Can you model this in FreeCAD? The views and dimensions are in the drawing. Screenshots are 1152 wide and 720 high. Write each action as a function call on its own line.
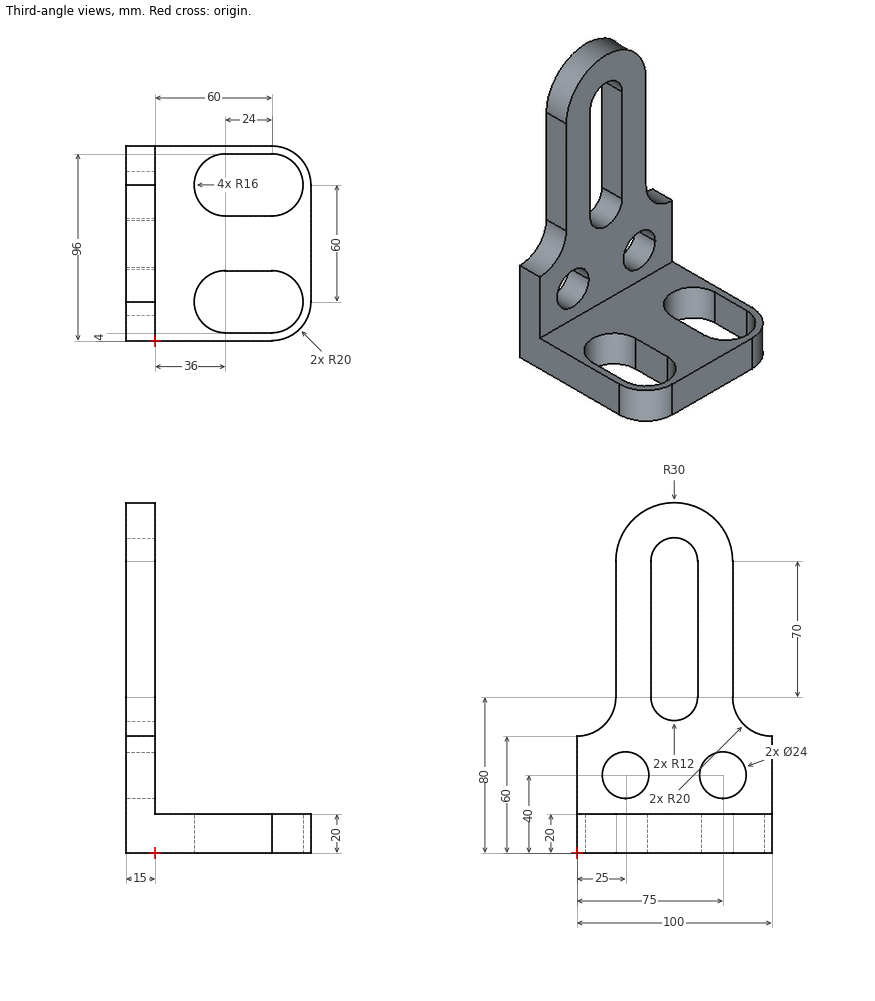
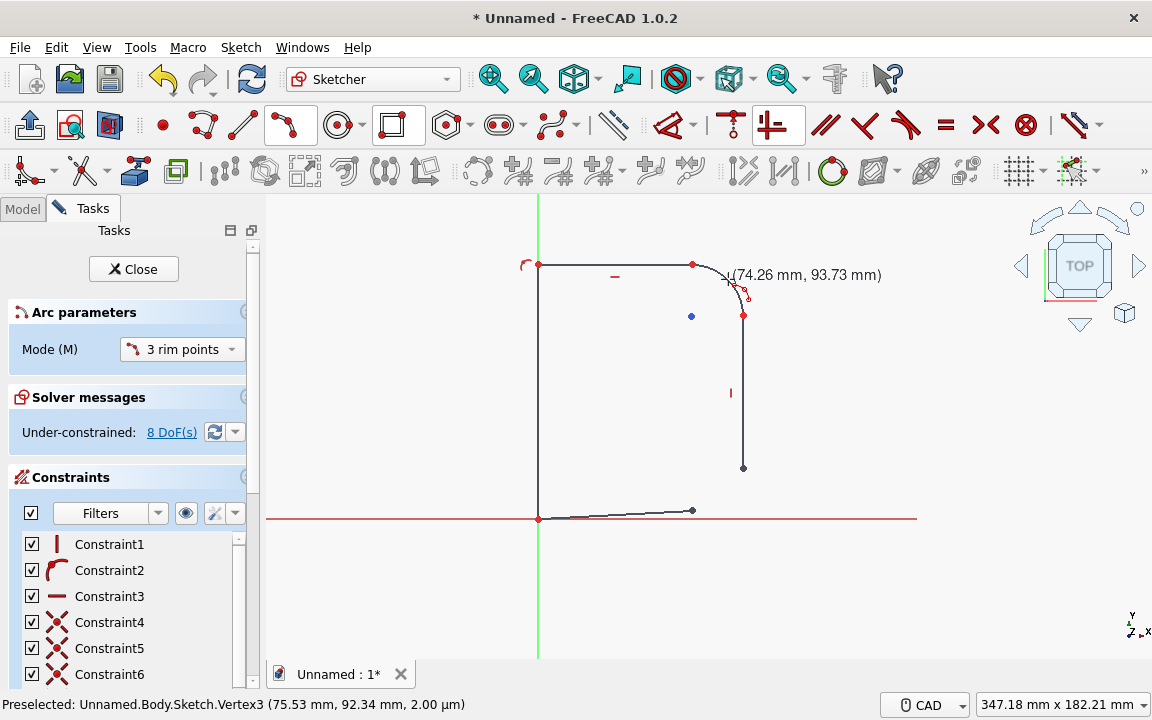
click(692, 511)
click(743, 469)
click(728, 504)
key(Escape)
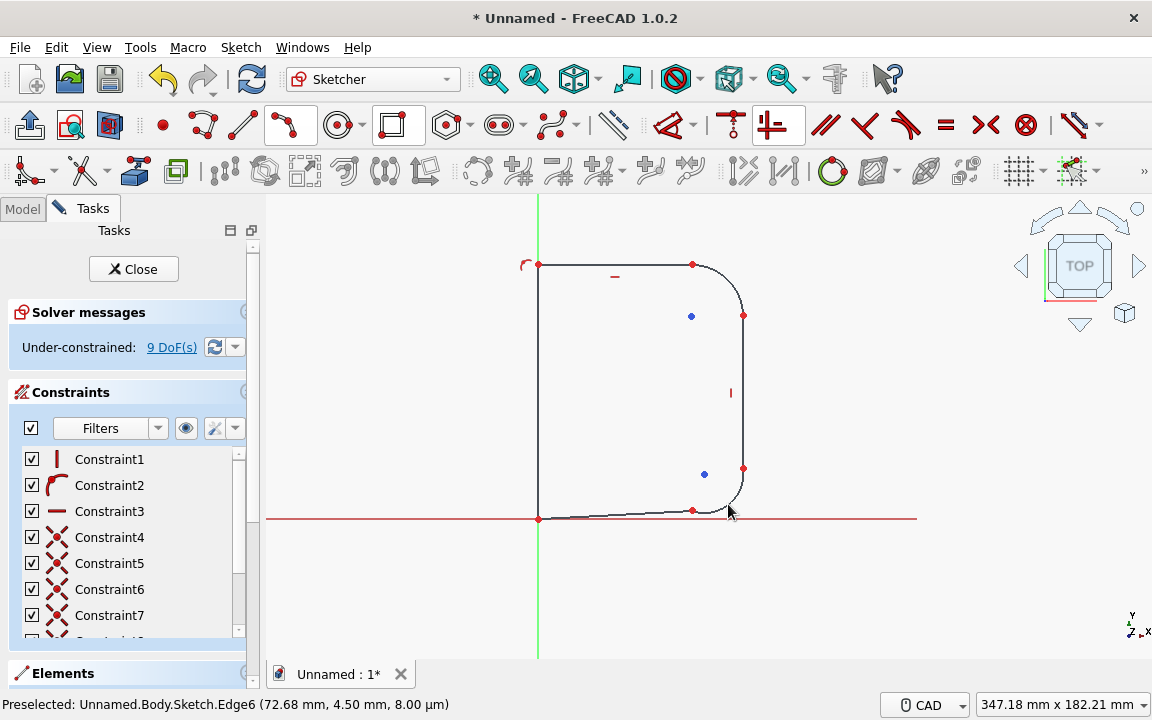
click(743, 423)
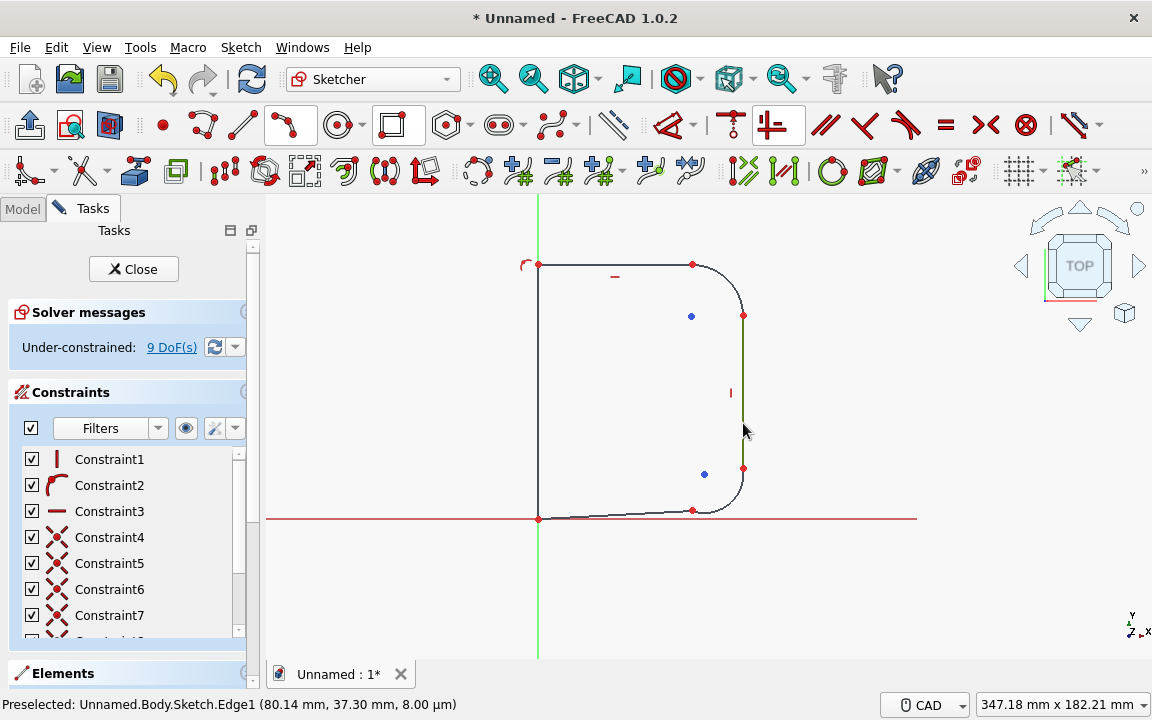
click(737, 293)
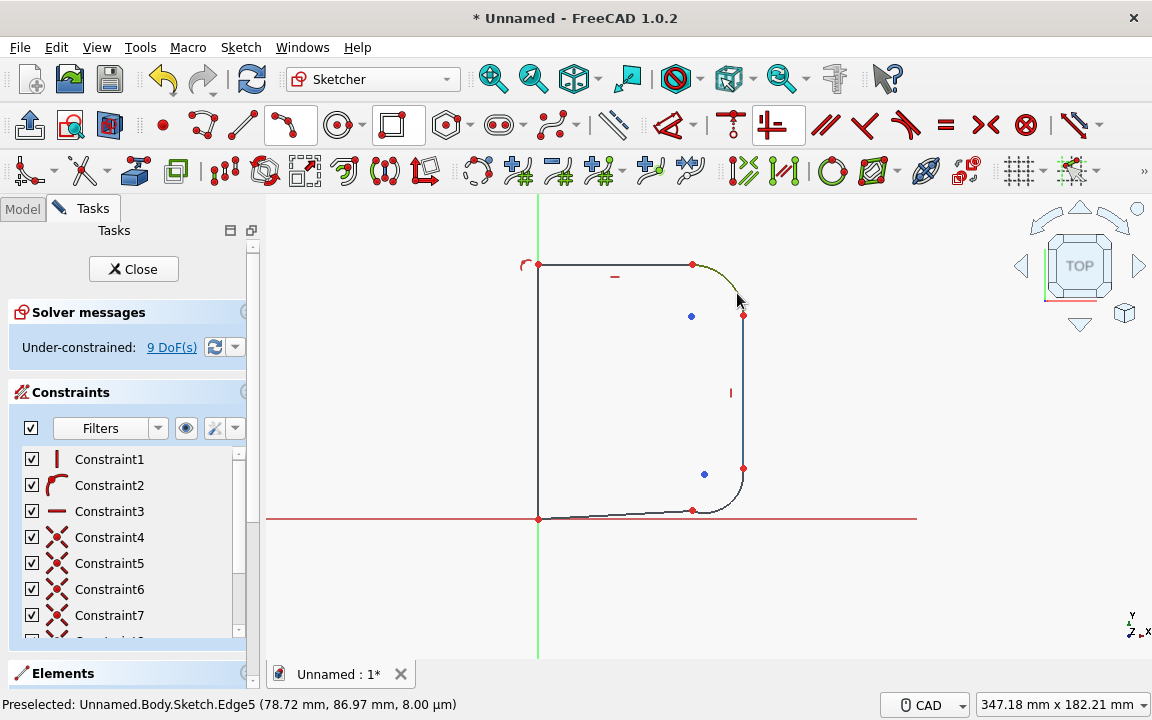
click(906, 126)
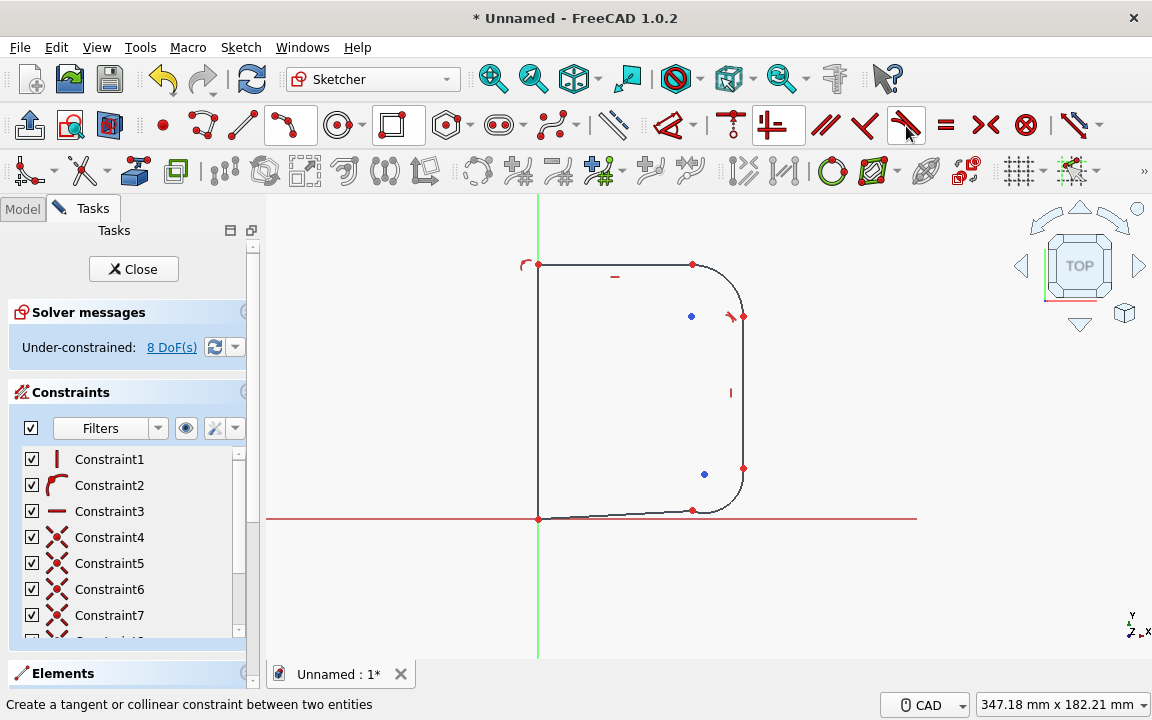
click(743, 423)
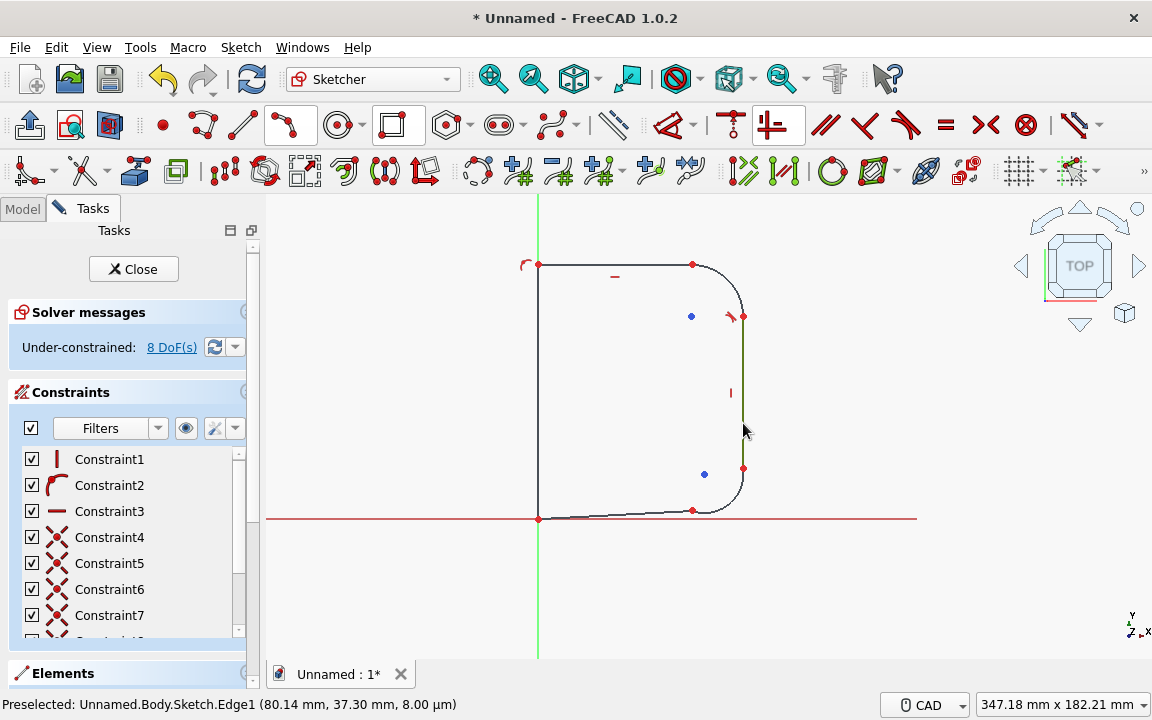
click(739, 492)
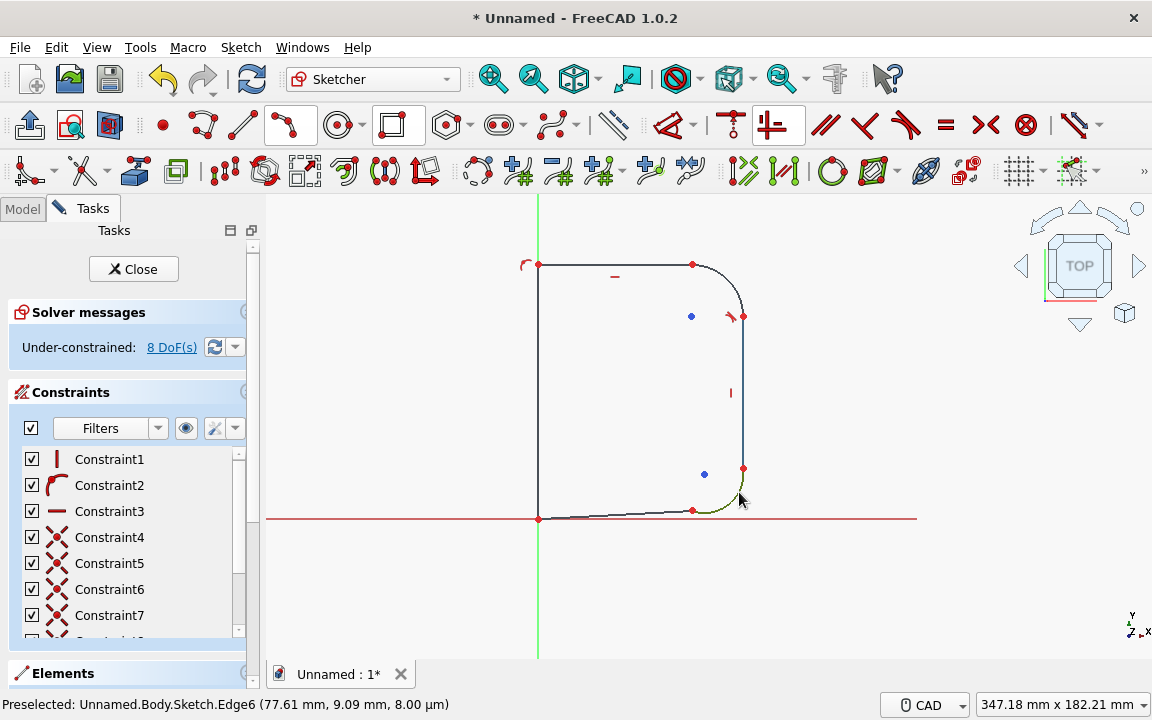
click(906, 126)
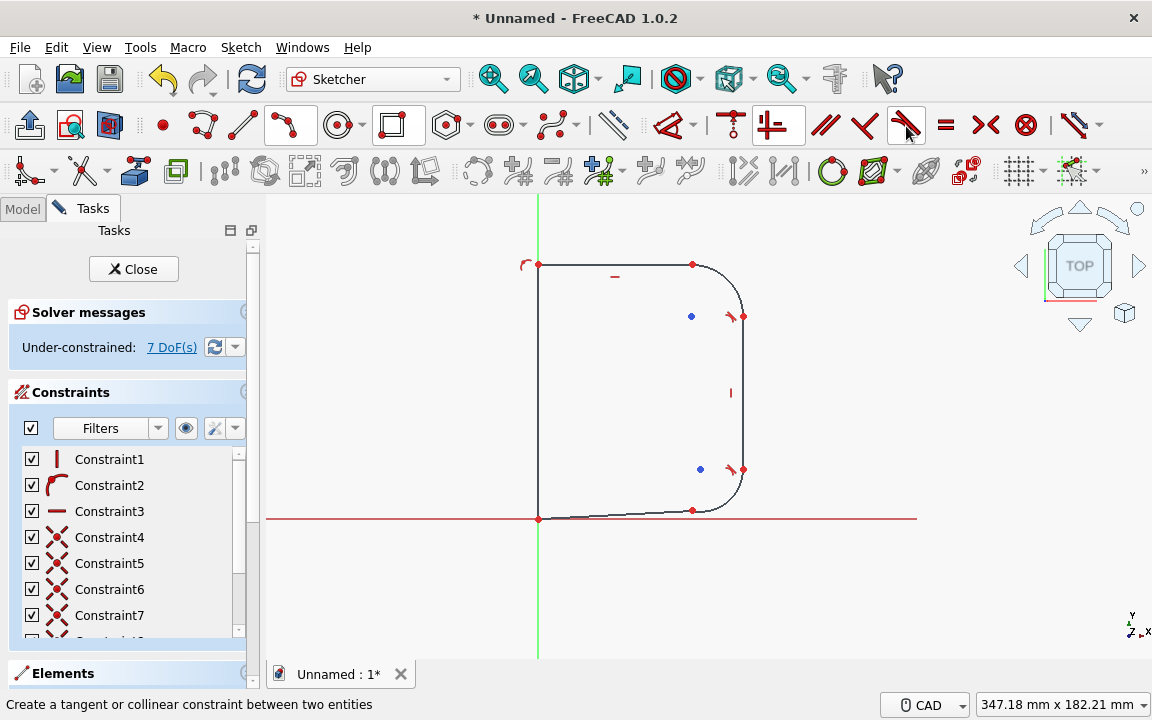
click(646, 265)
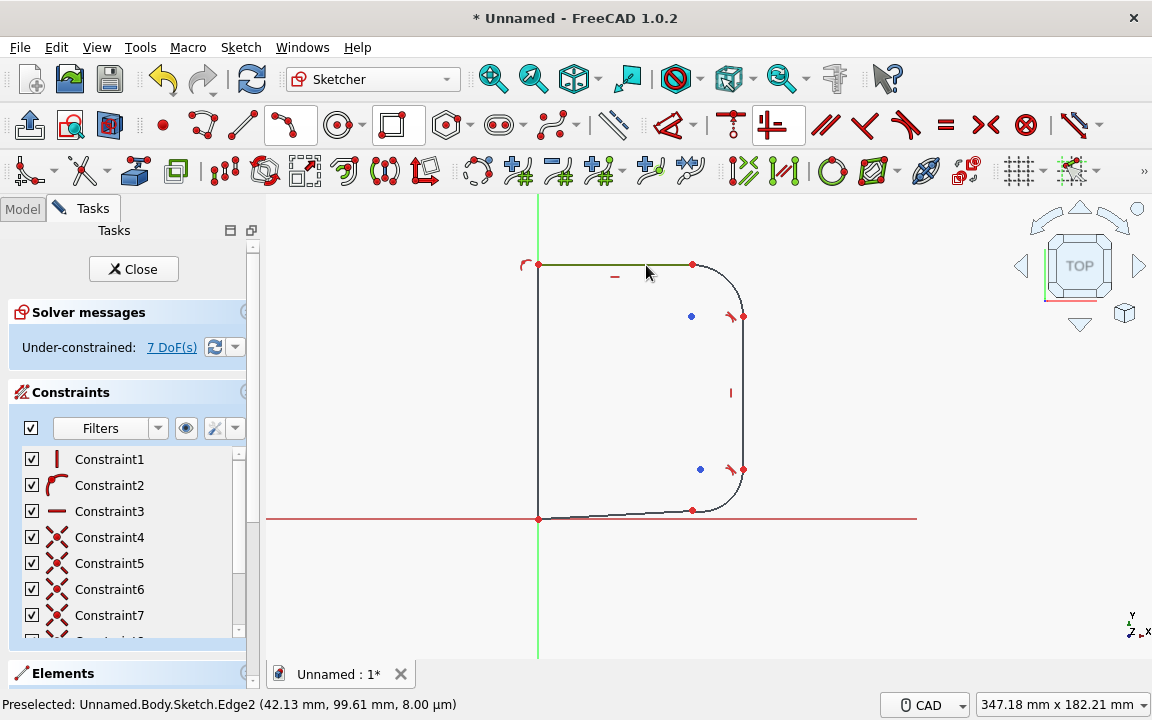
click(737, 293)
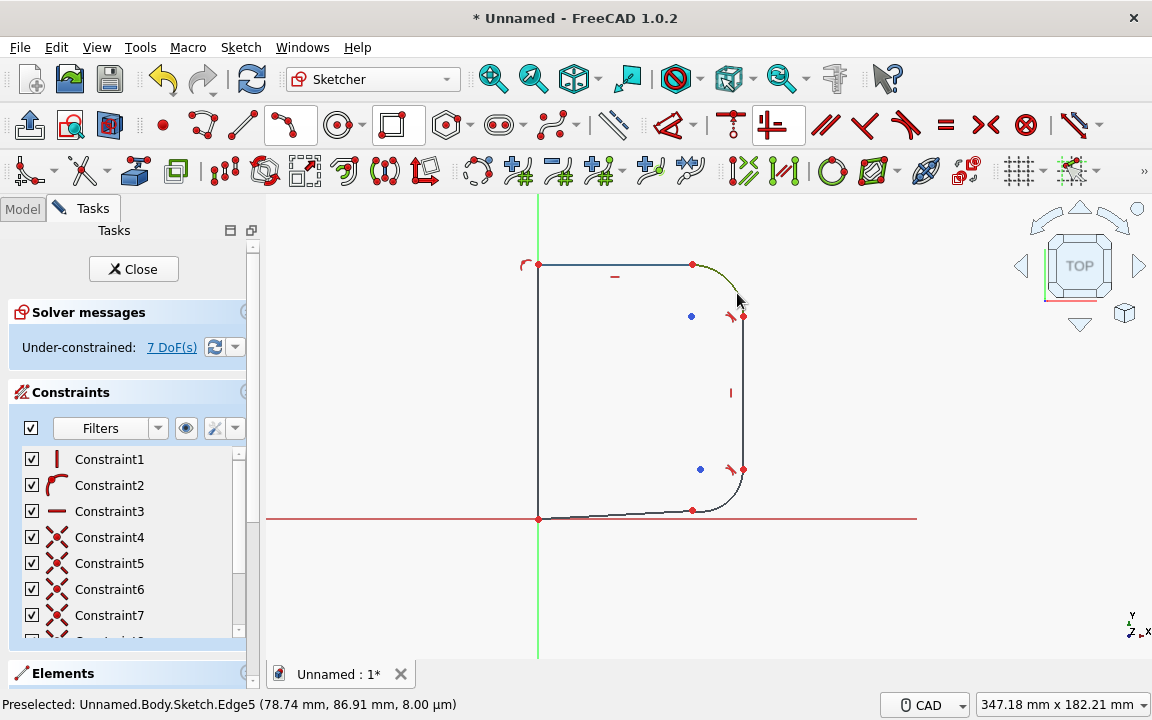
click(906, 126)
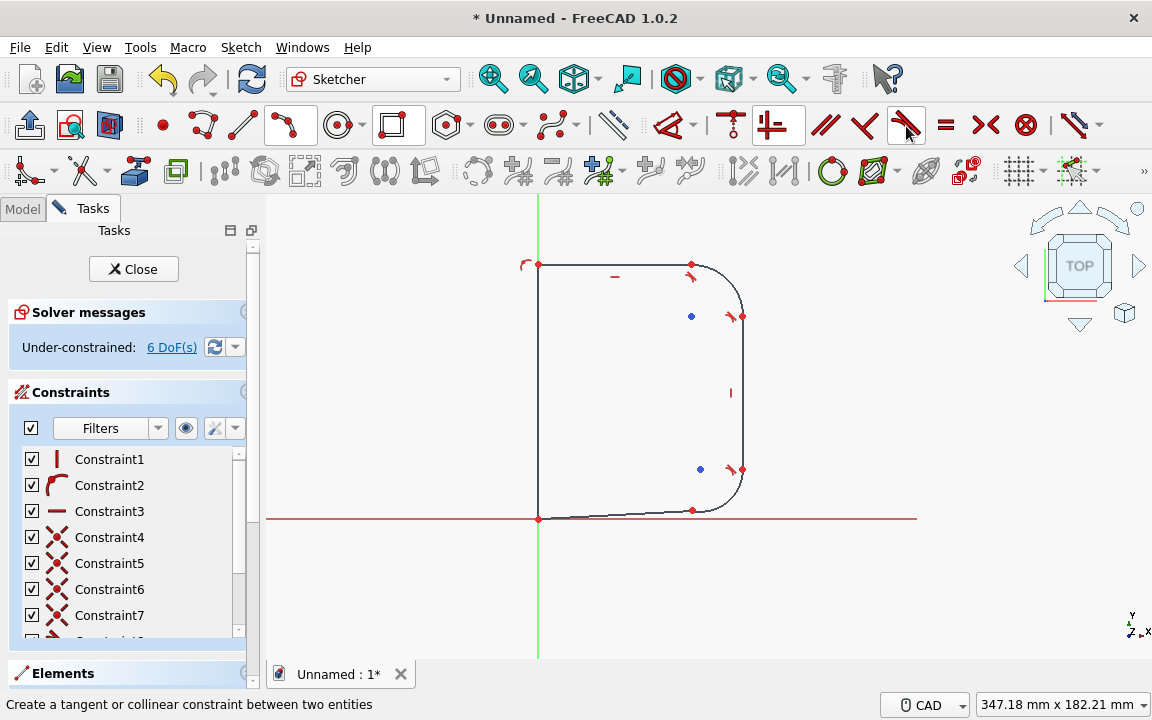
click(585, 517)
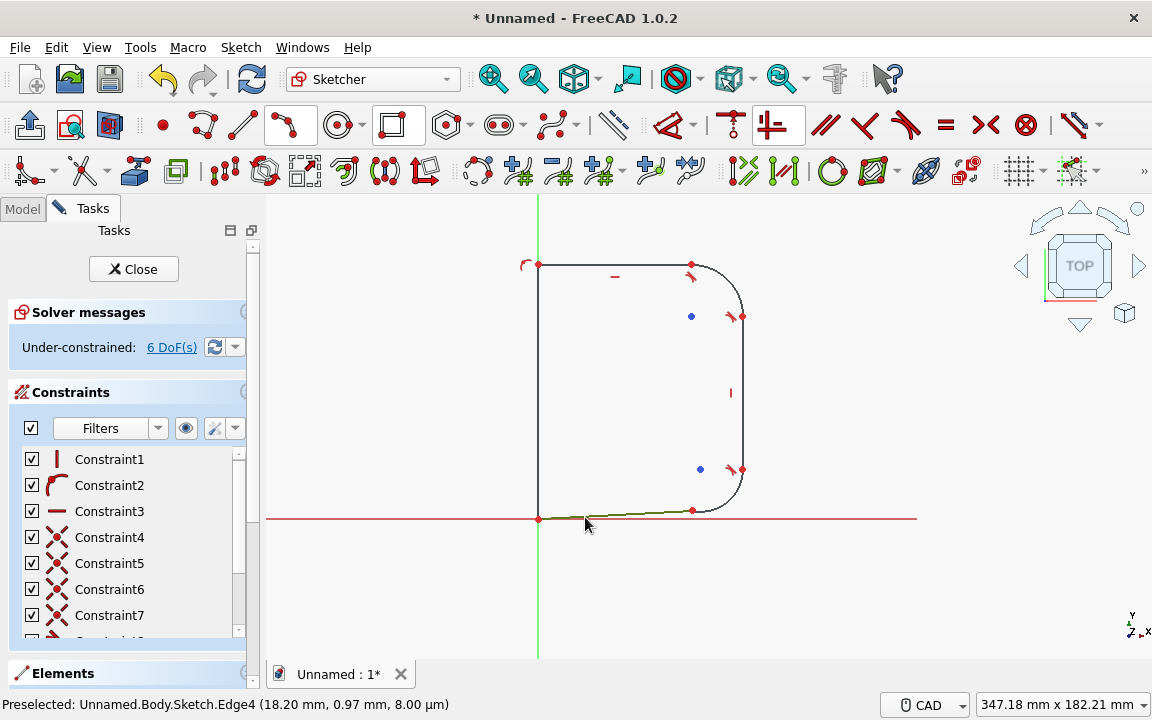
scroll(714, 509, up, 2)